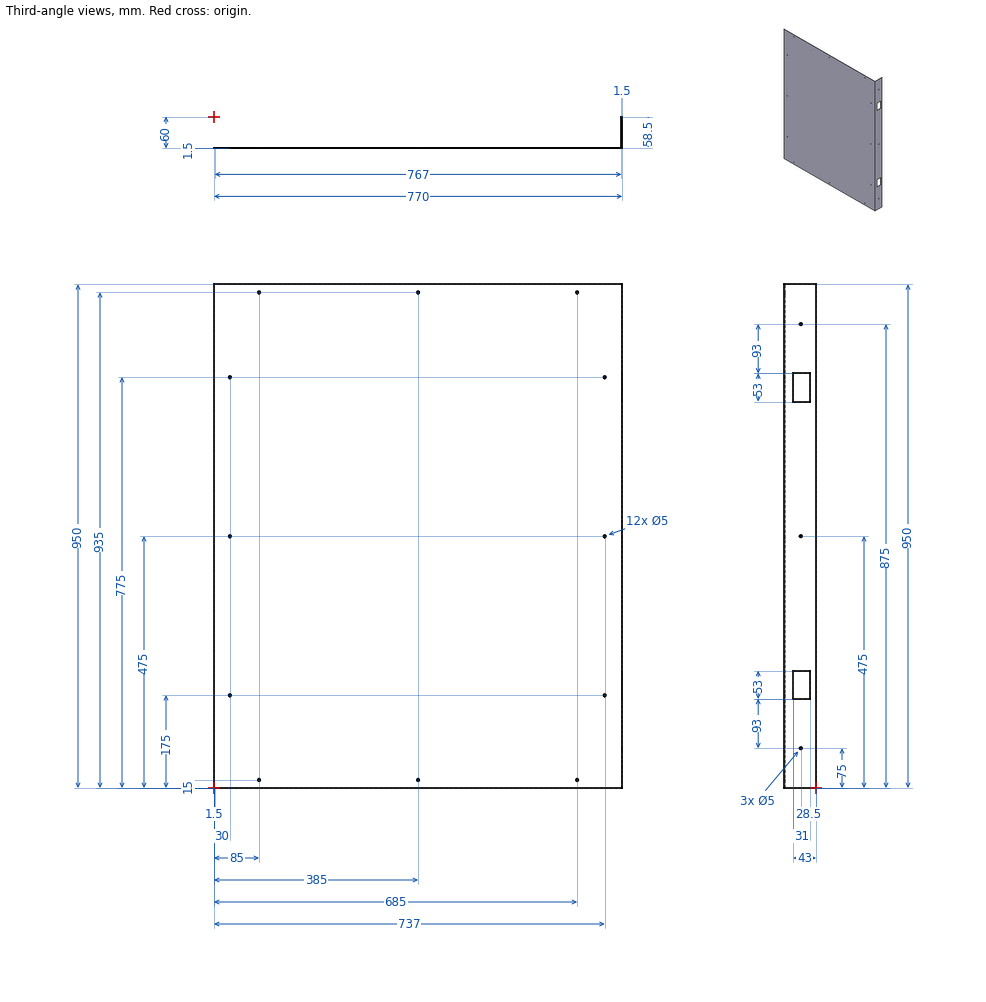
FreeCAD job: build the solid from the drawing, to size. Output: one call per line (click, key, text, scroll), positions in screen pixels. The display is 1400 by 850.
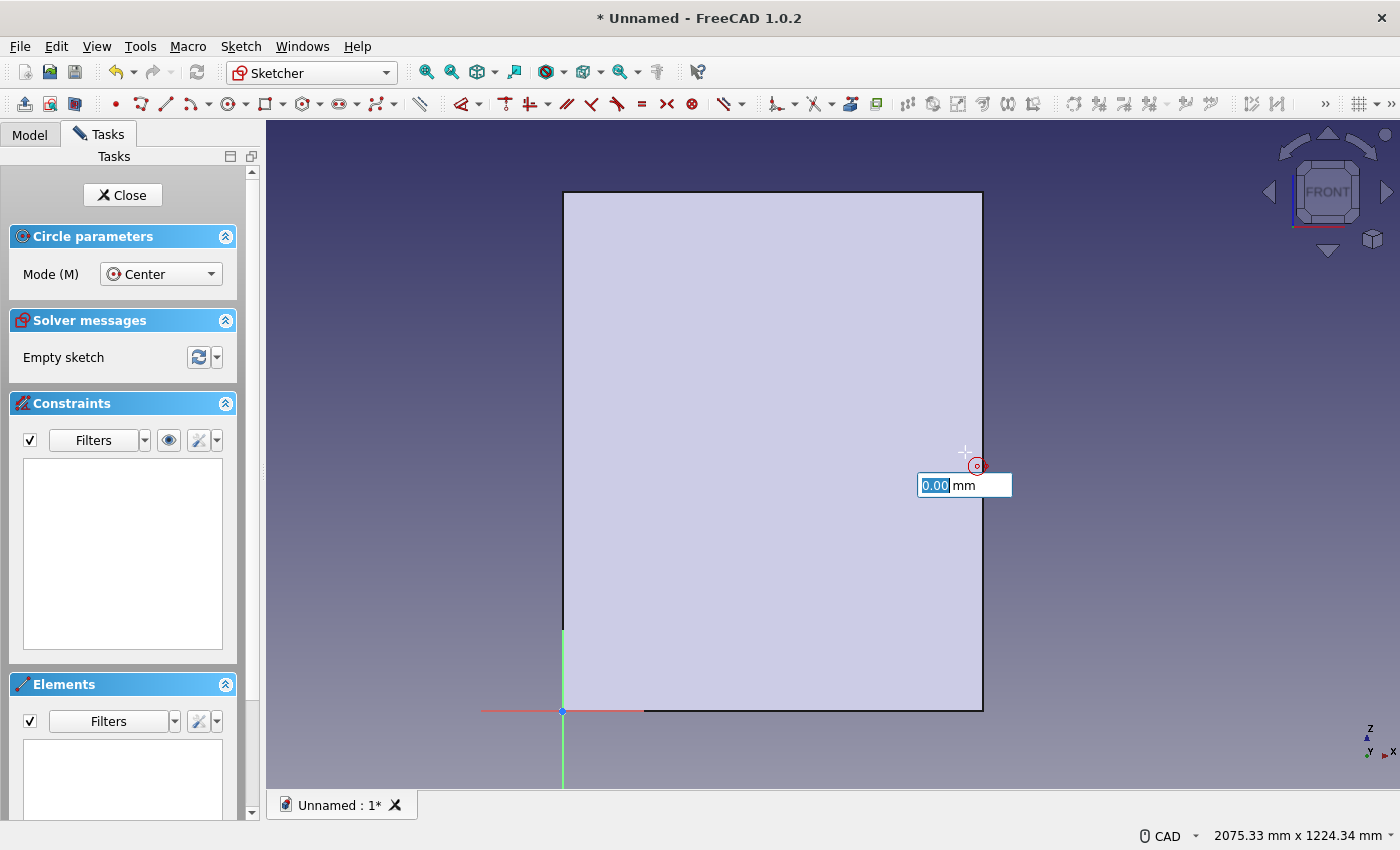
scroll(966, 451, up, 13)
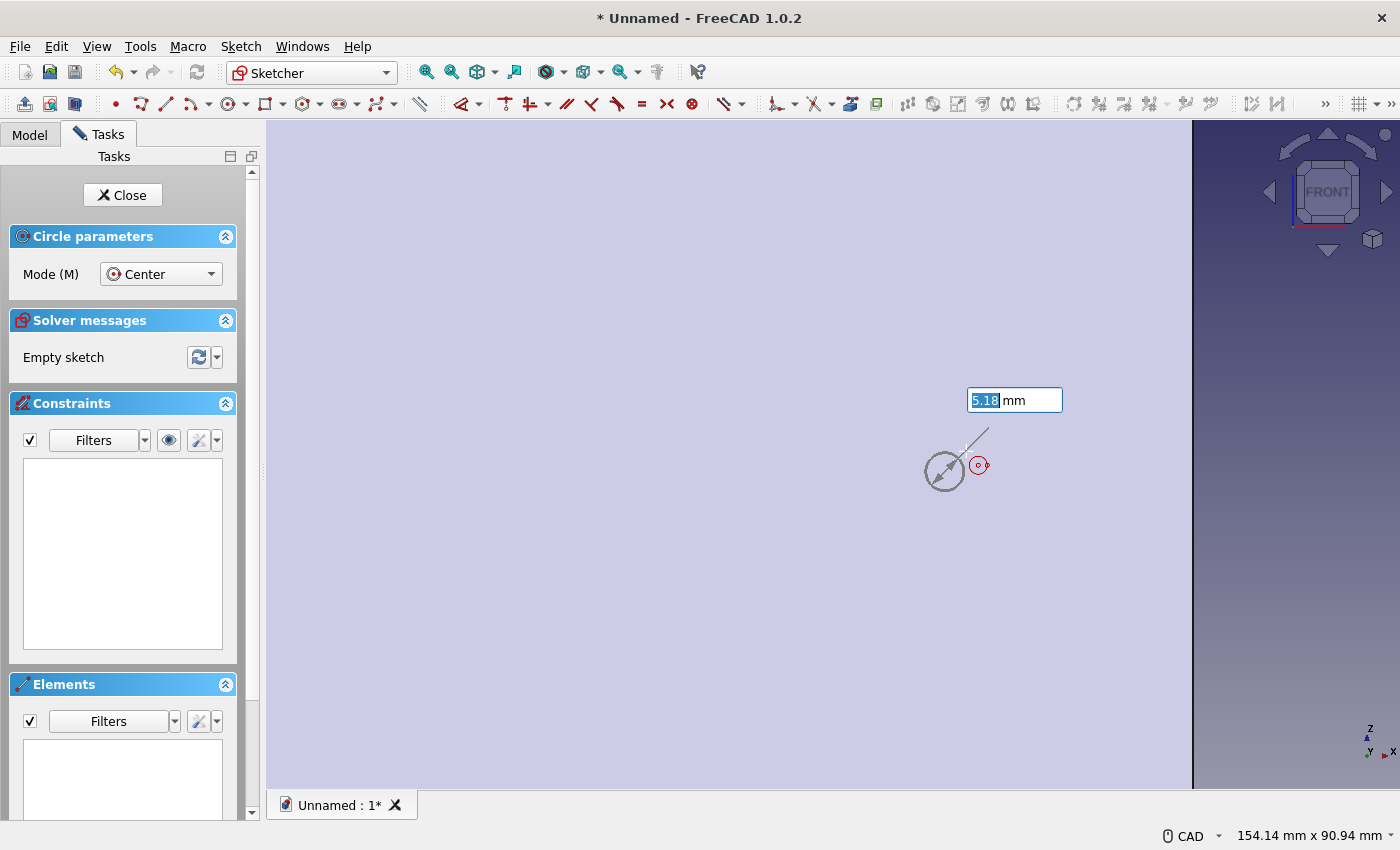
click(964, 441)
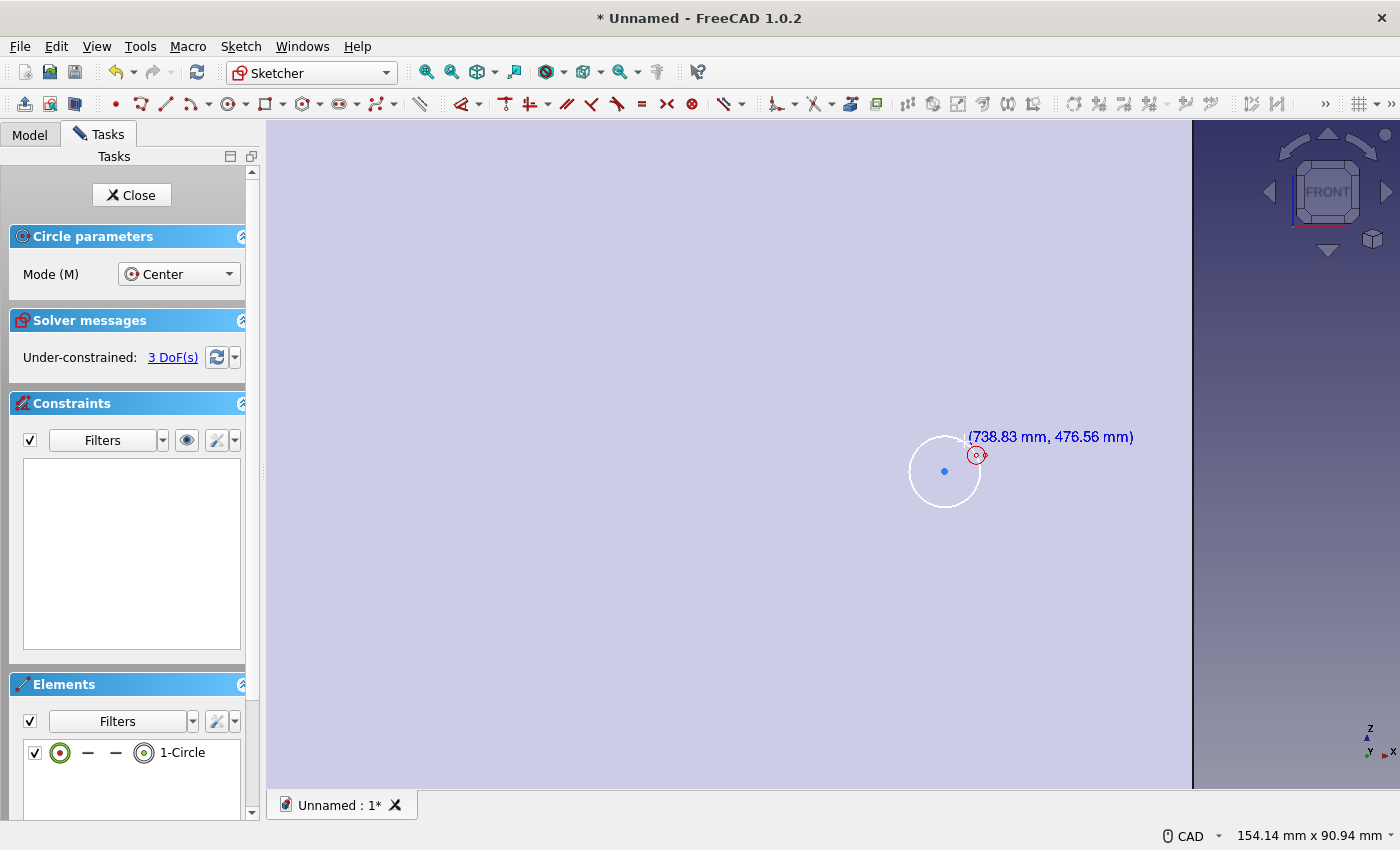
scroll(927, 452, down, 14)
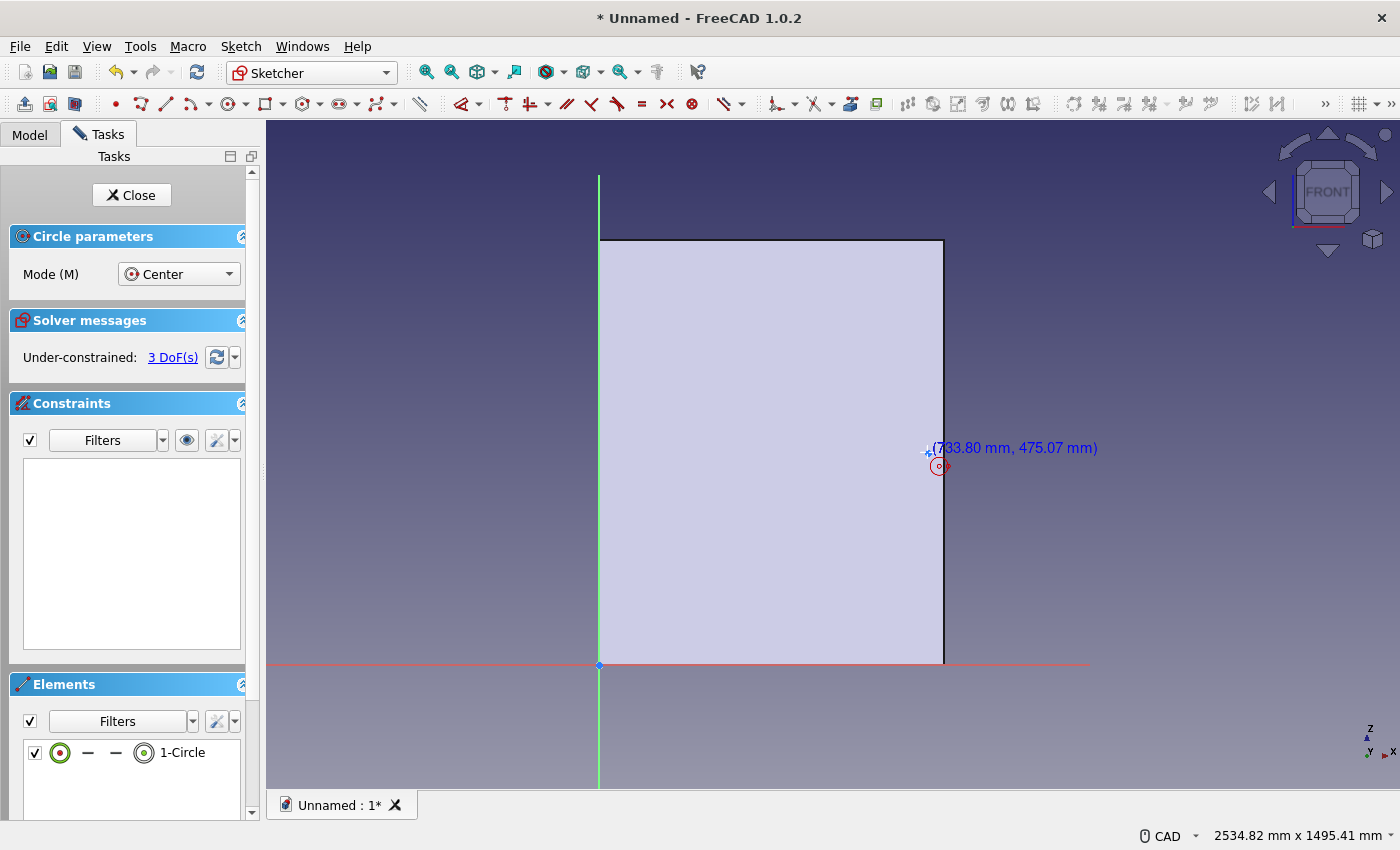
scroll(929, 318, up, 16)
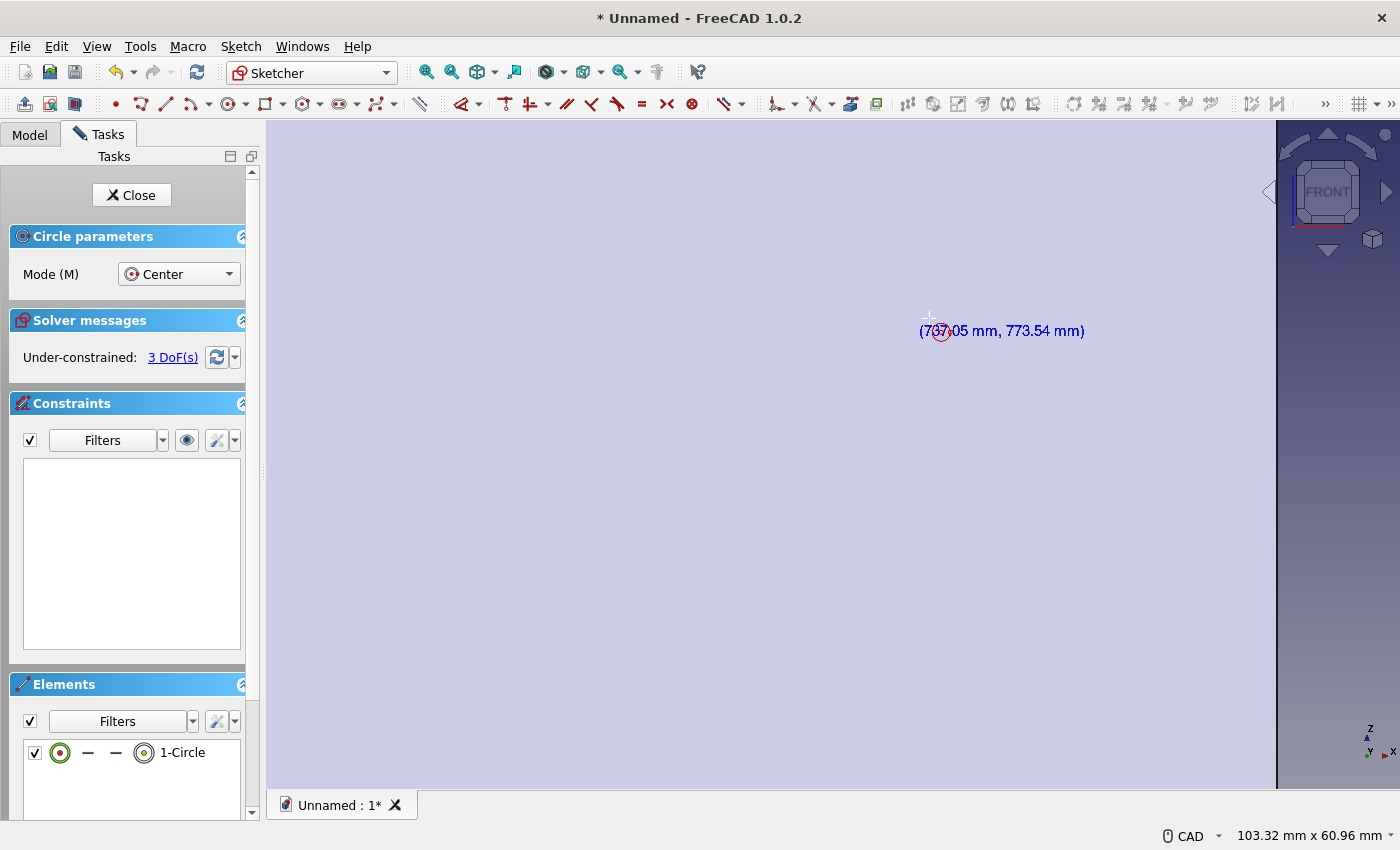
scroll(968, 285, down, 15)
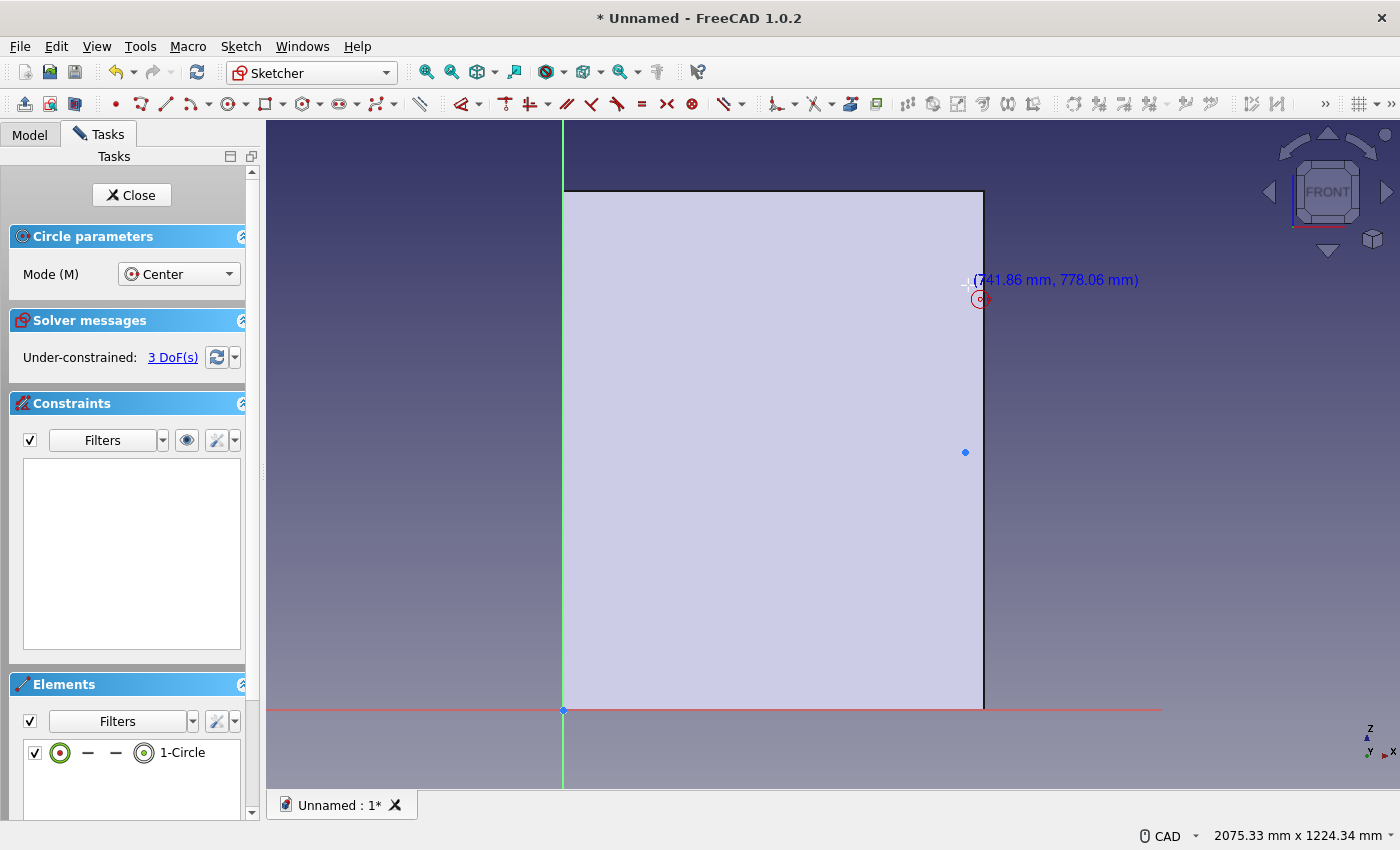
click(966, 287)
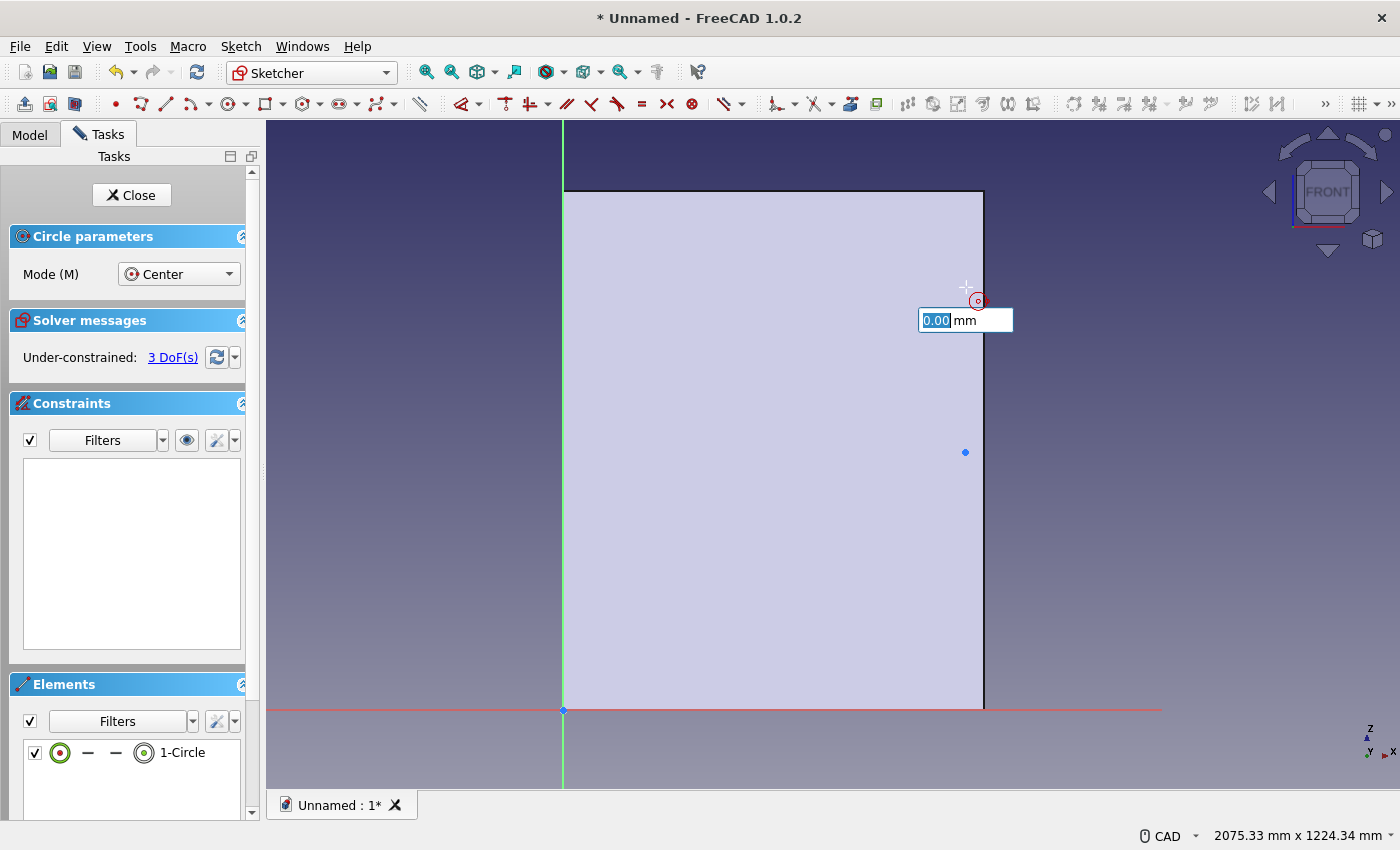
scroll(967, 286, up, 13)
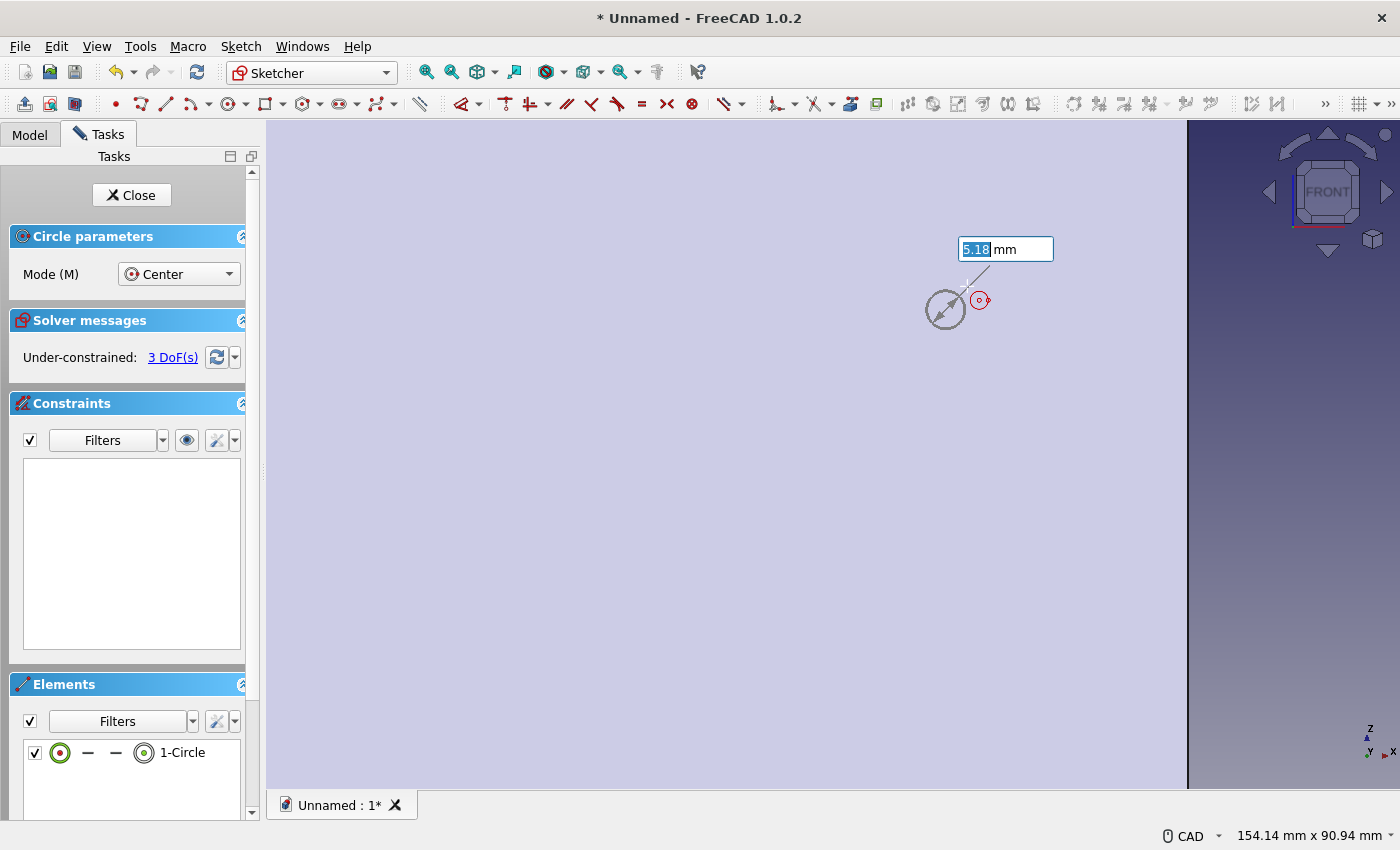
click(958, 283)